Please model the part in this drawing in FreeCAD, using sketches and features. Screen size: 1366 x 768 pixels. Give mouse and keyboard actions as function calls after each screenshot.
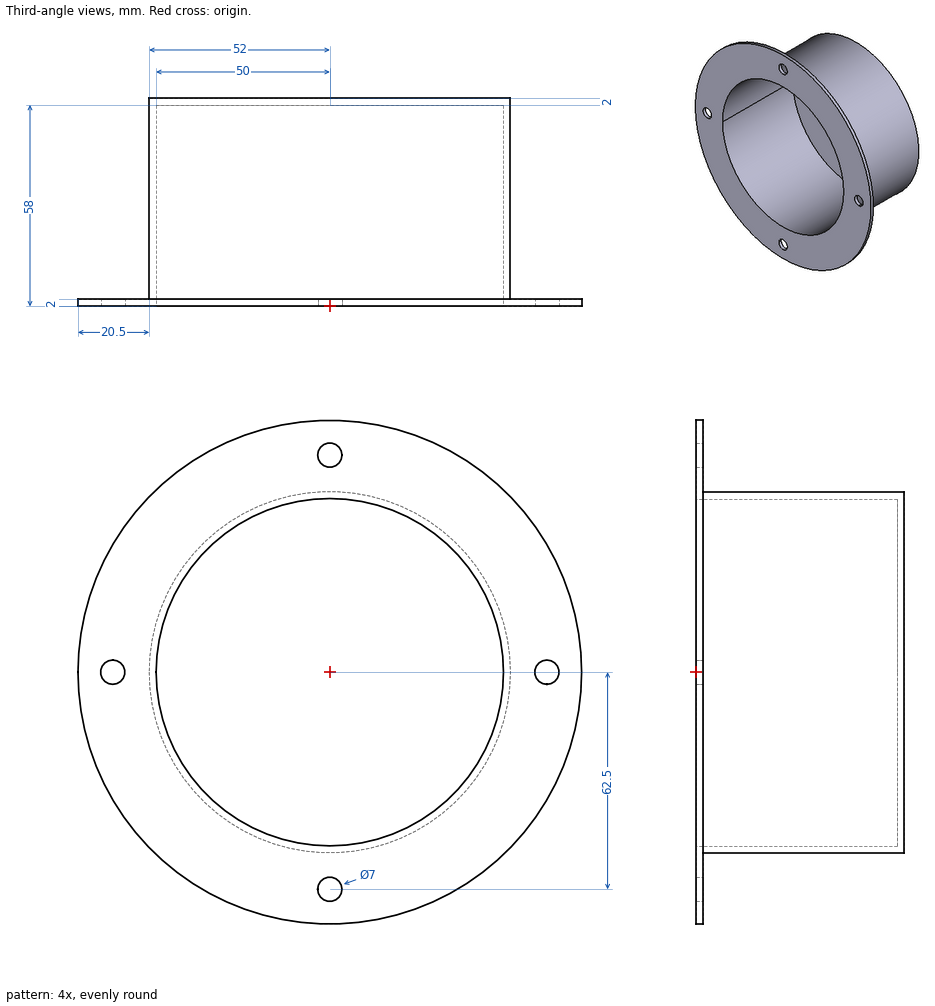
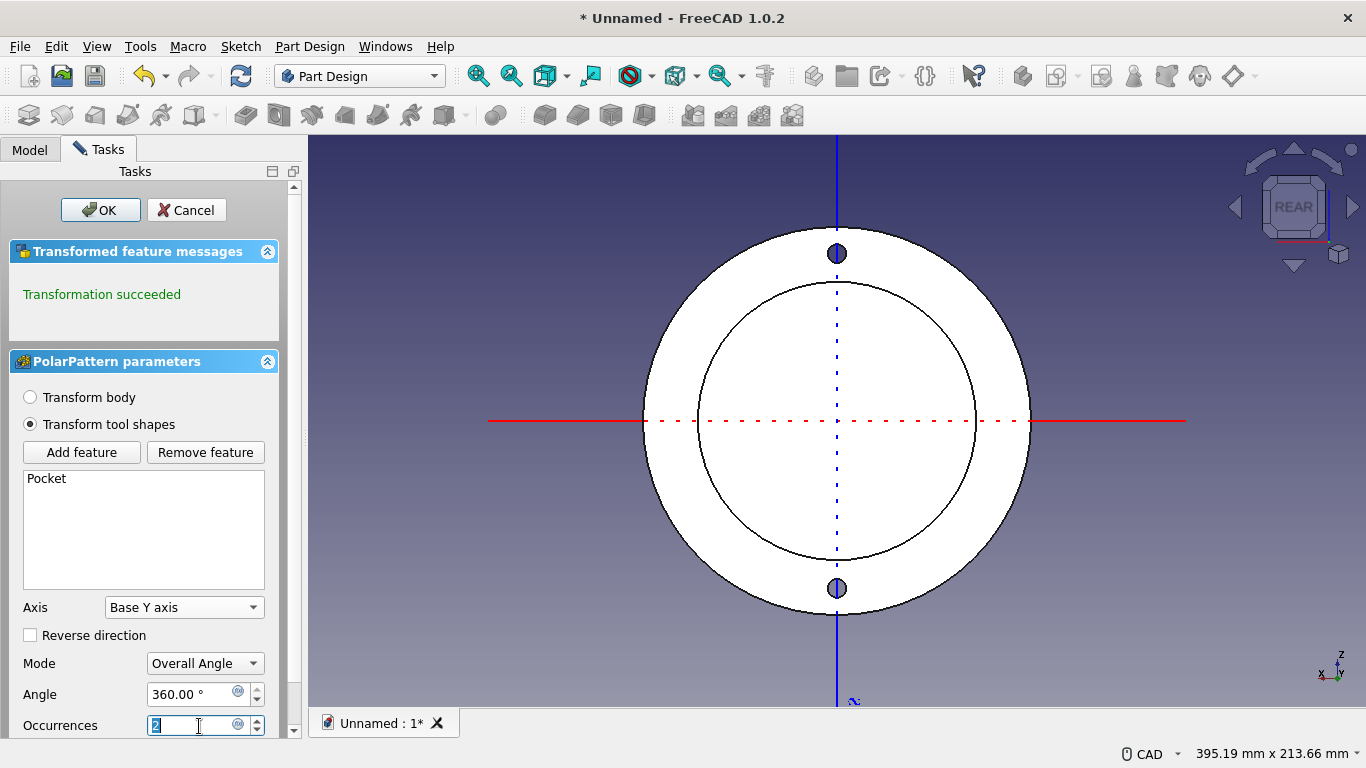
text(4)
key(Tab)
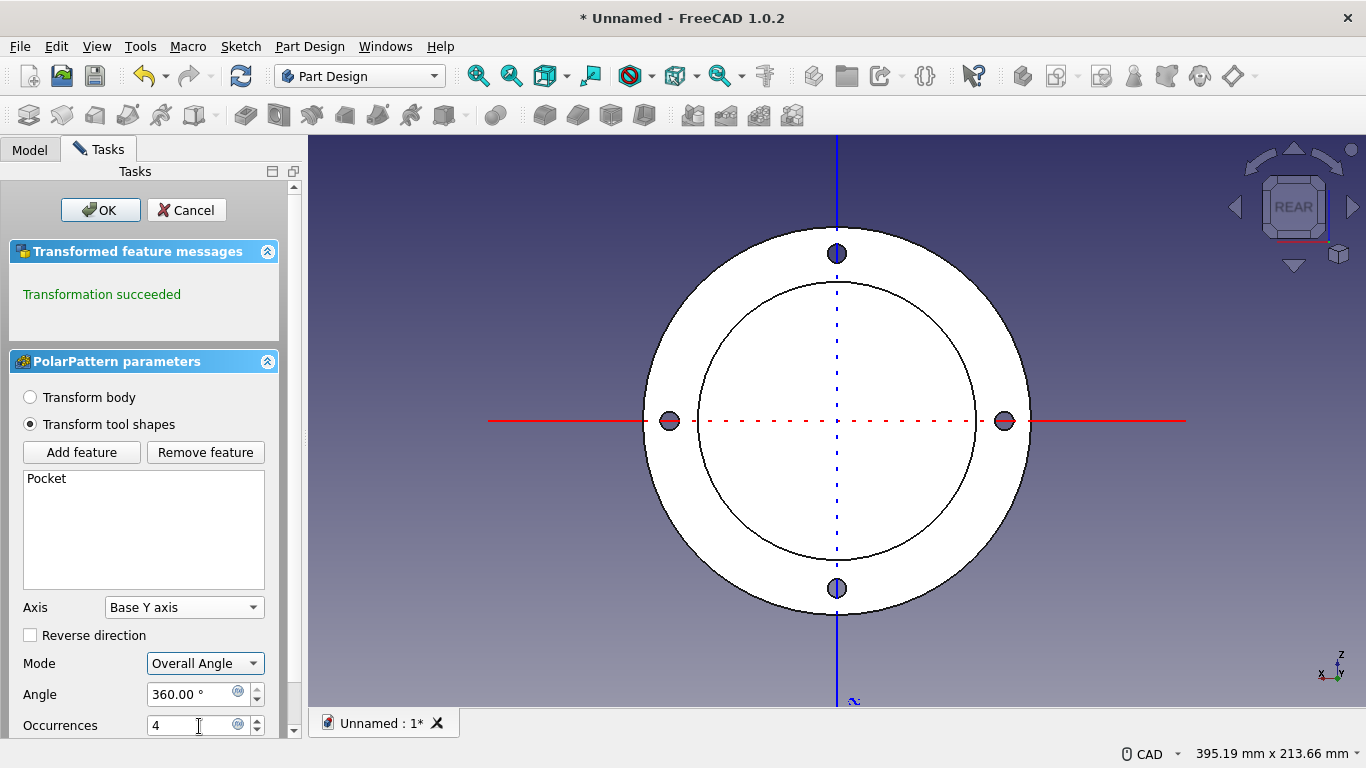
click(101, 210)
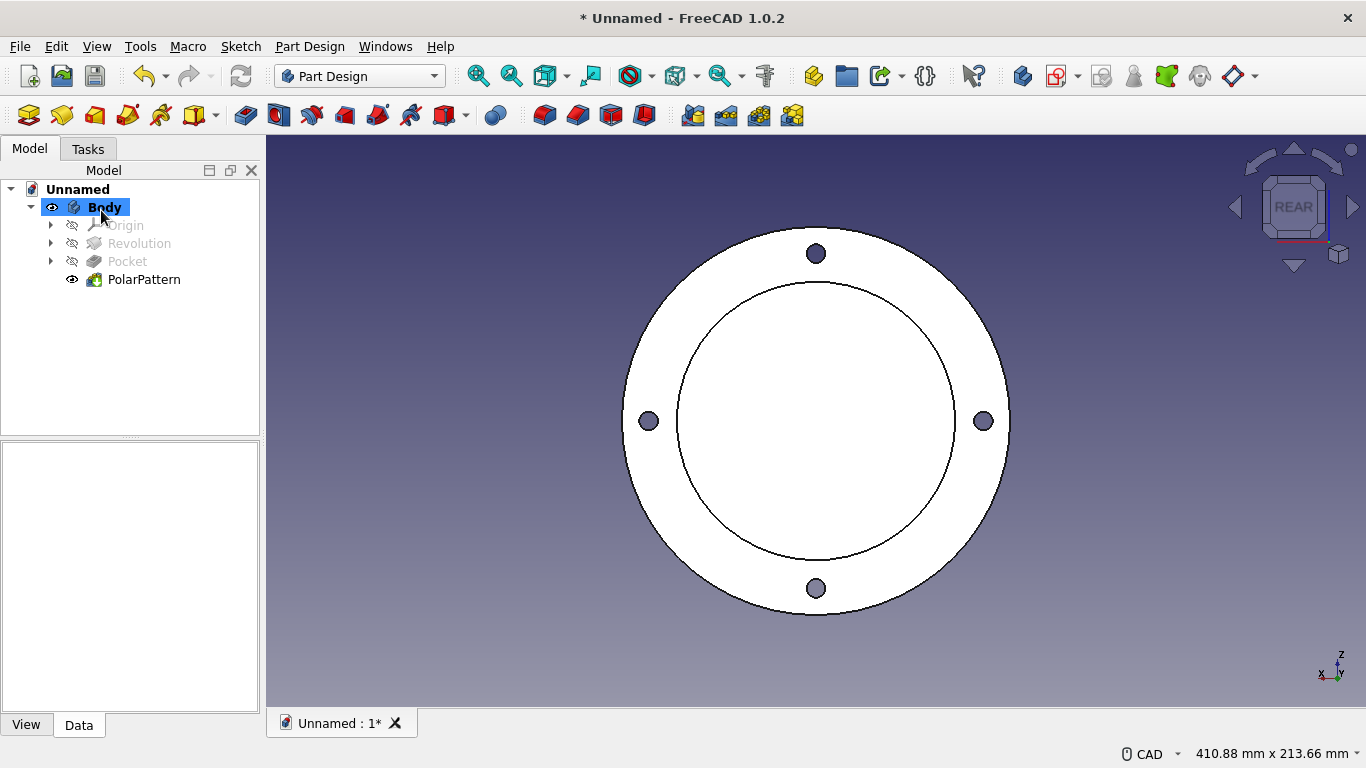
key(0)